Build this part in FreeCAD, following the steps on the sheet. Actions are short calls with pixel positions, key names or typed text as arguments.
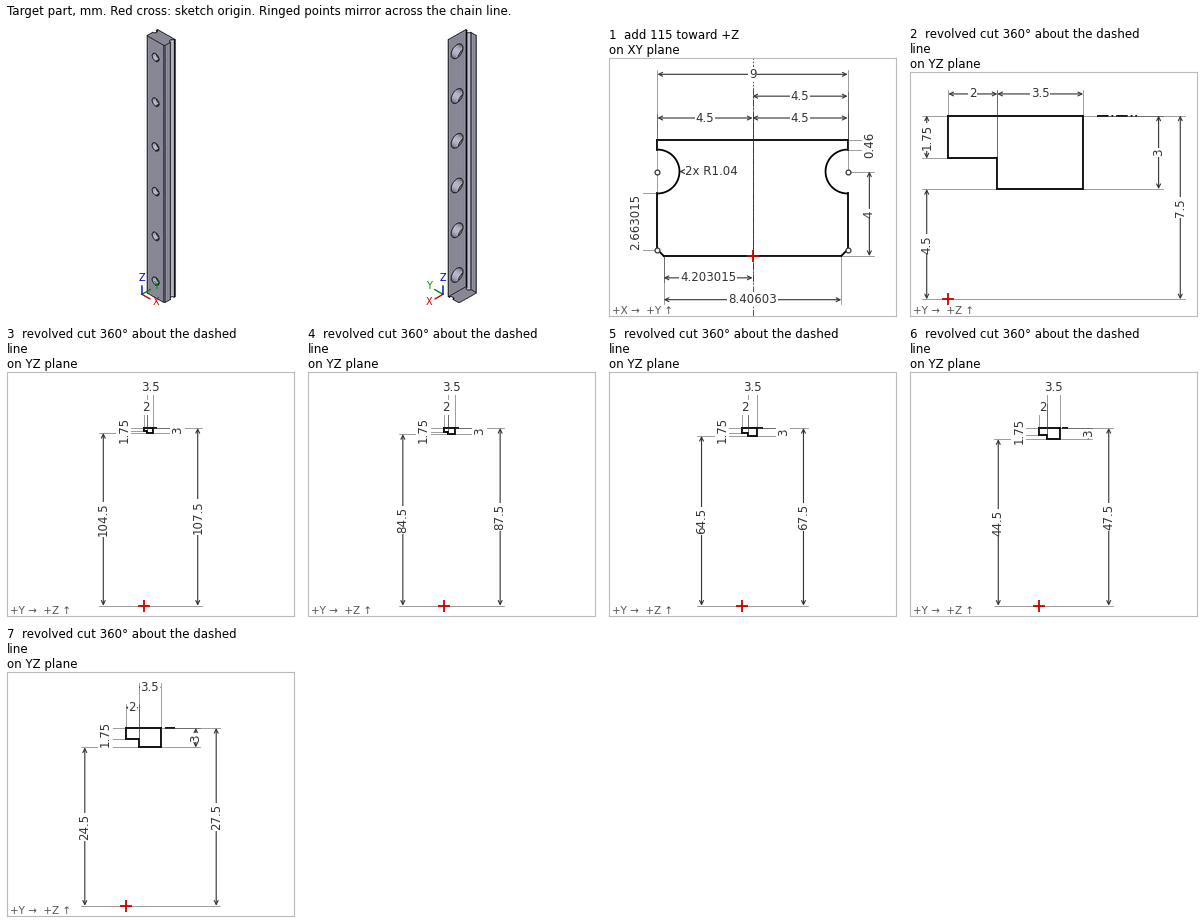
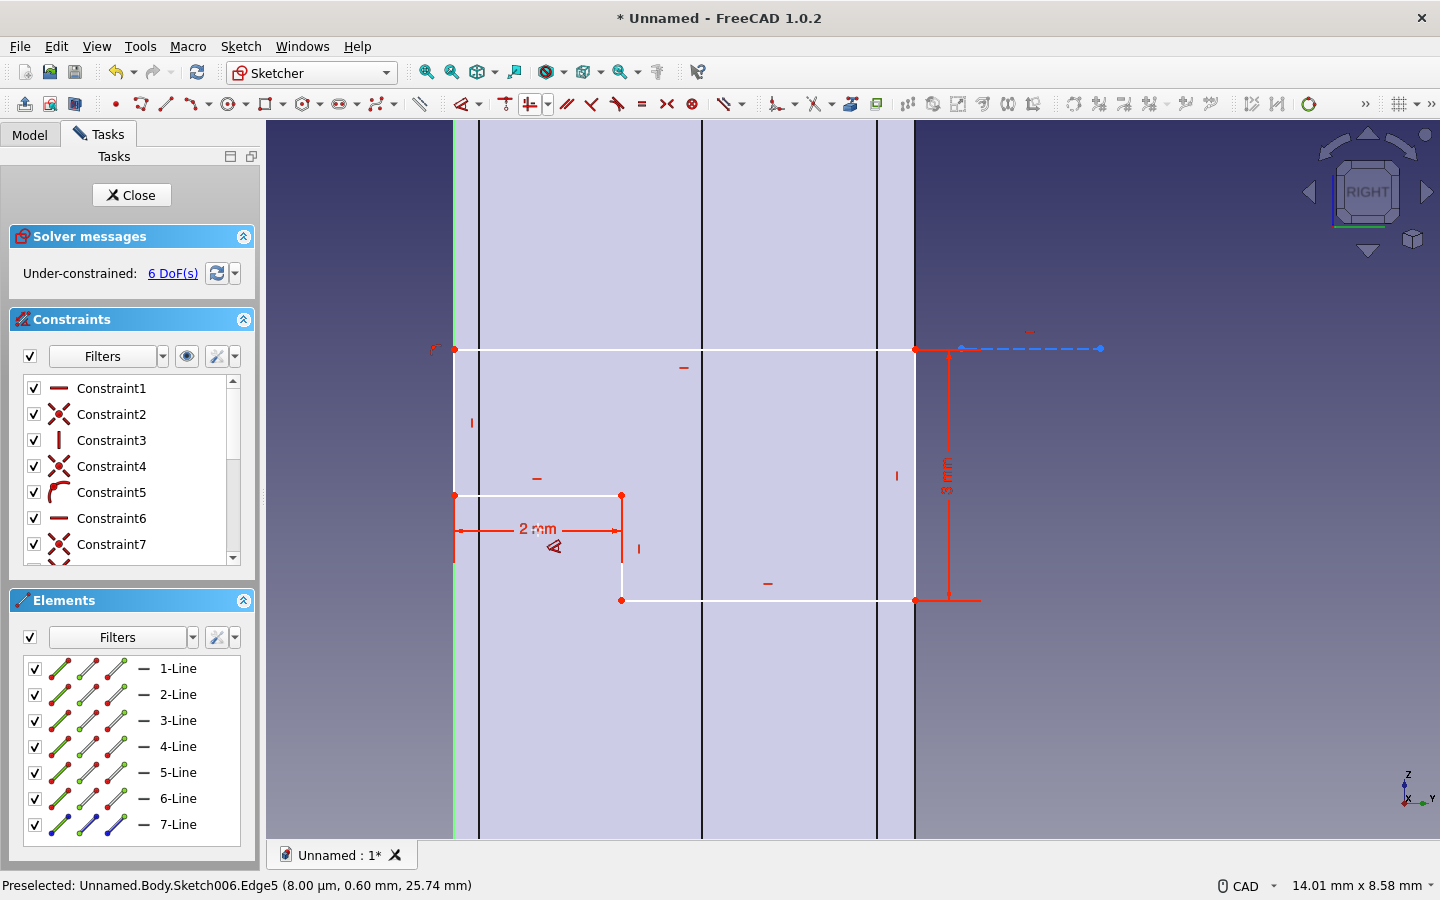
click(710, 601)
click(768, 635)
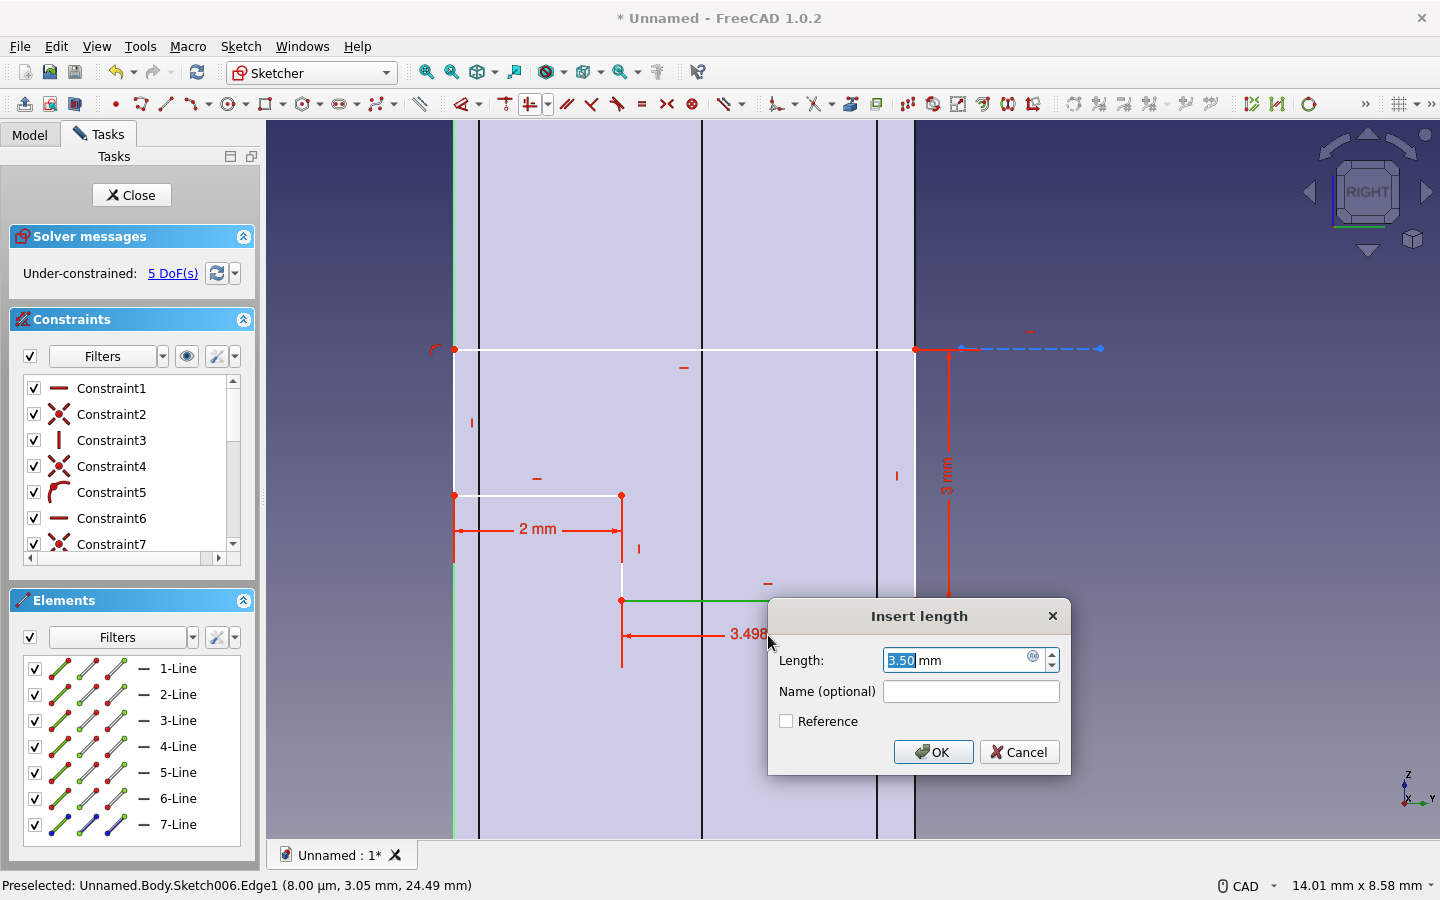
text(3.5)
key(Return)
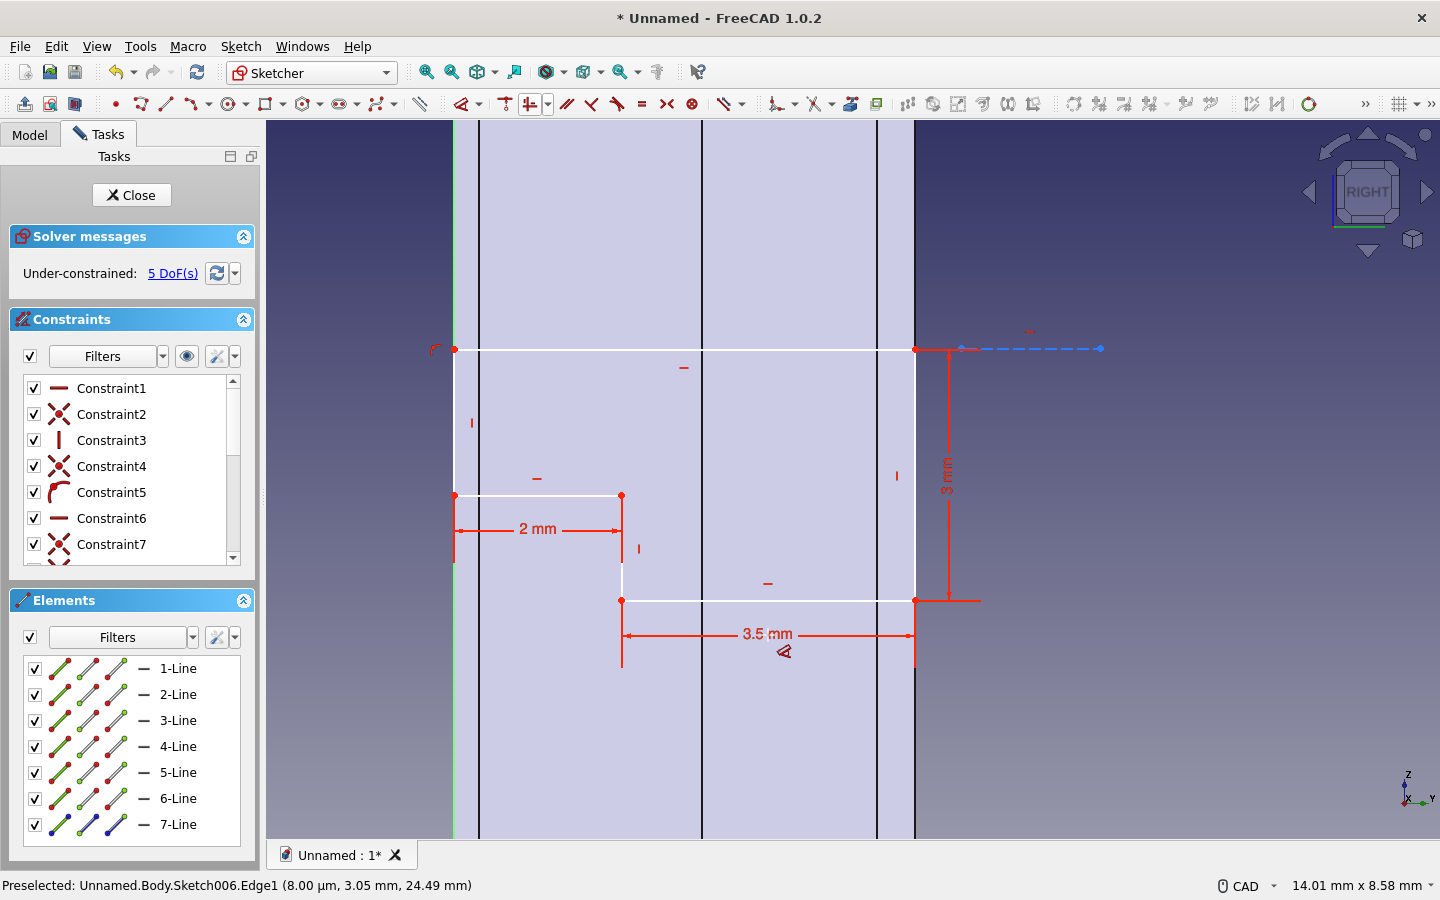
click(454, 393)
click(420, 423)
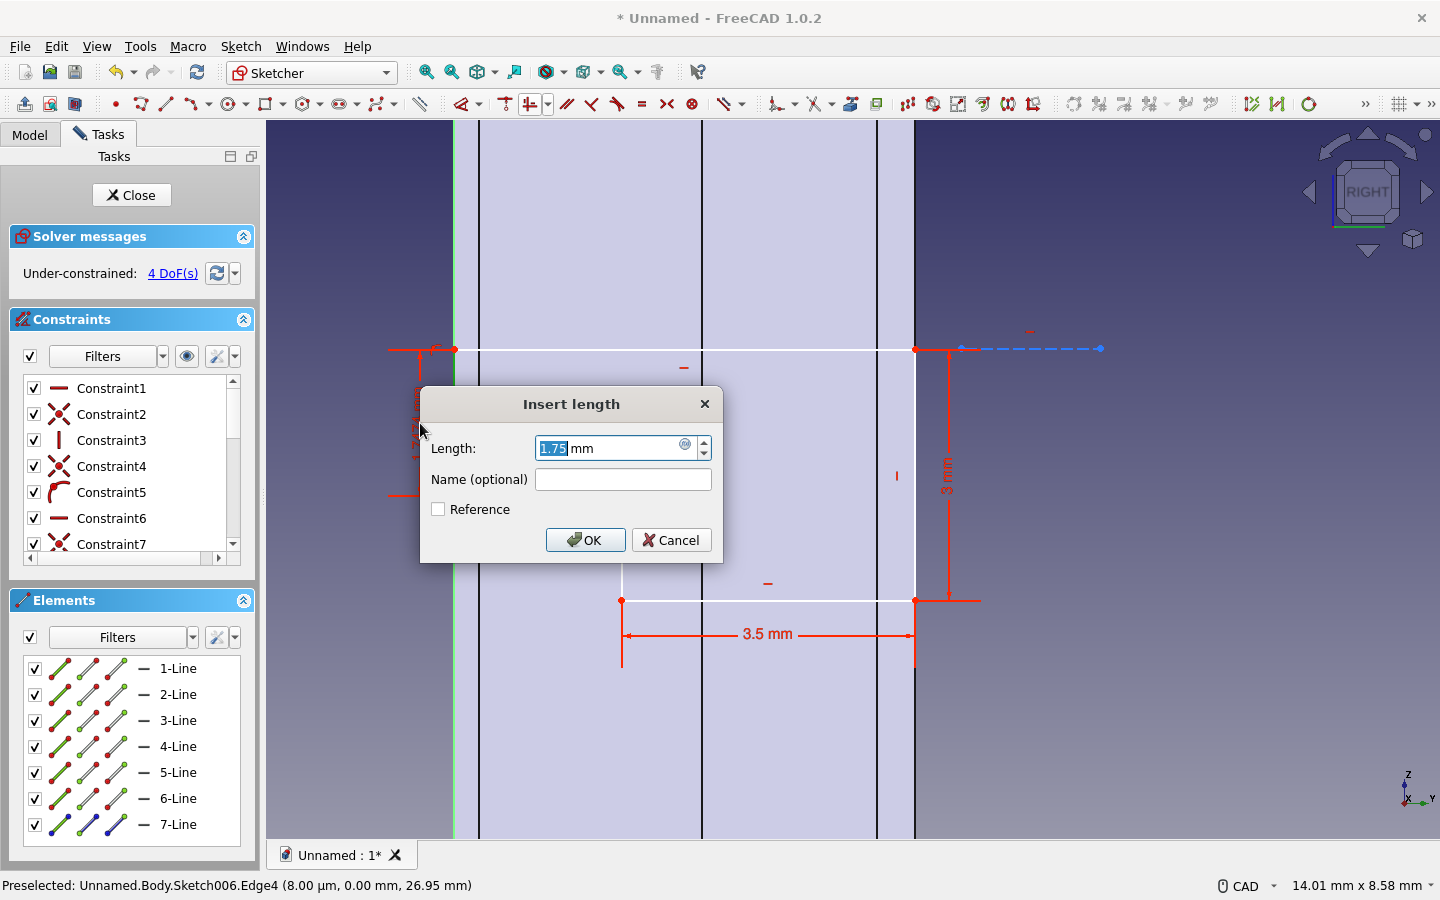
text(1.75)
key(Return)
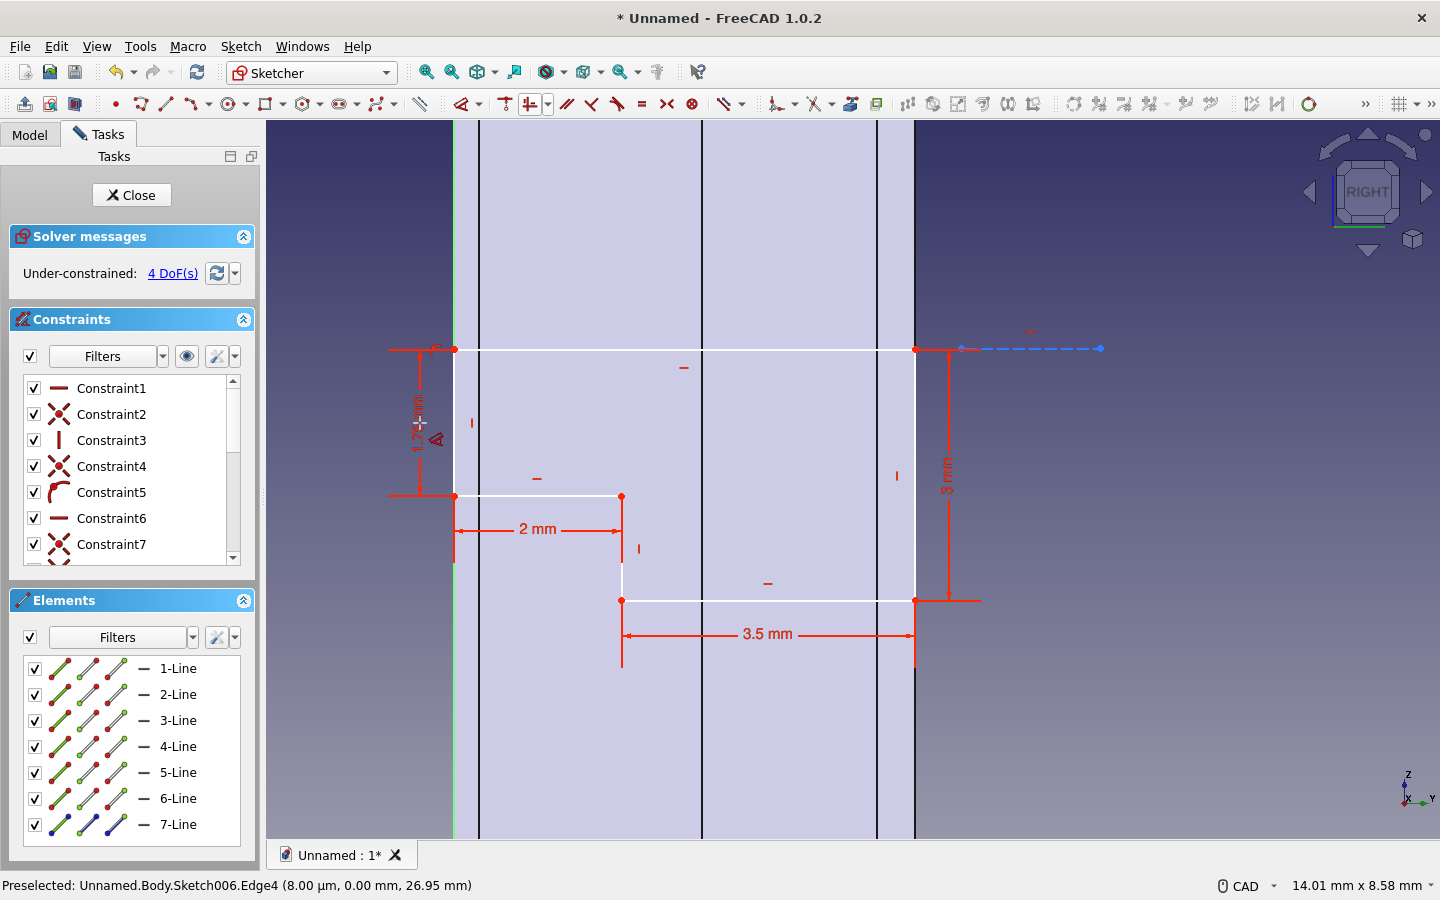
click(622, 601)
click(420, 706)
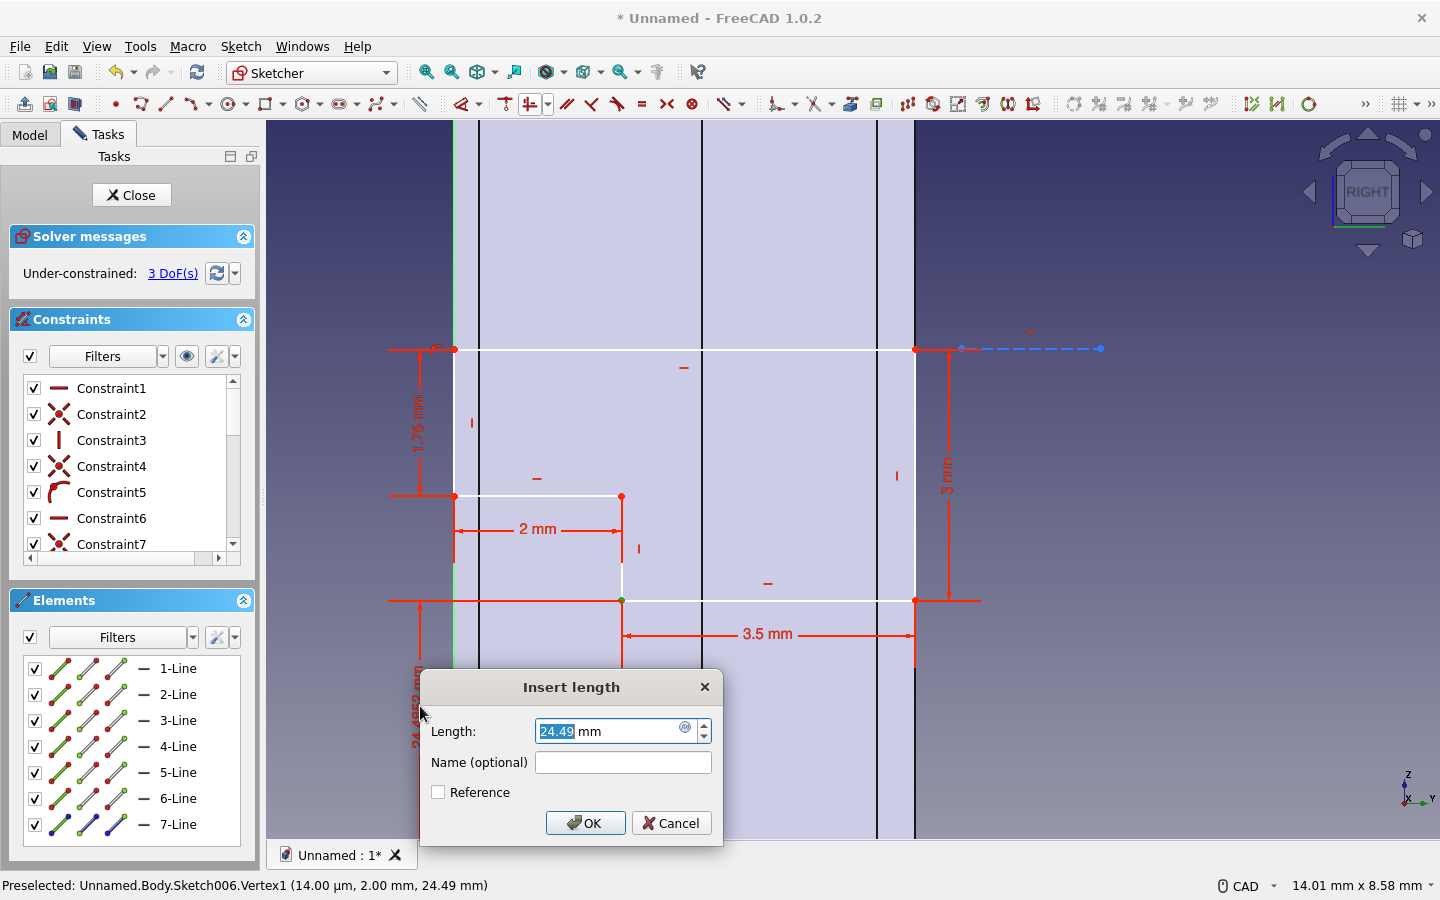
text(24.5)
key(Return)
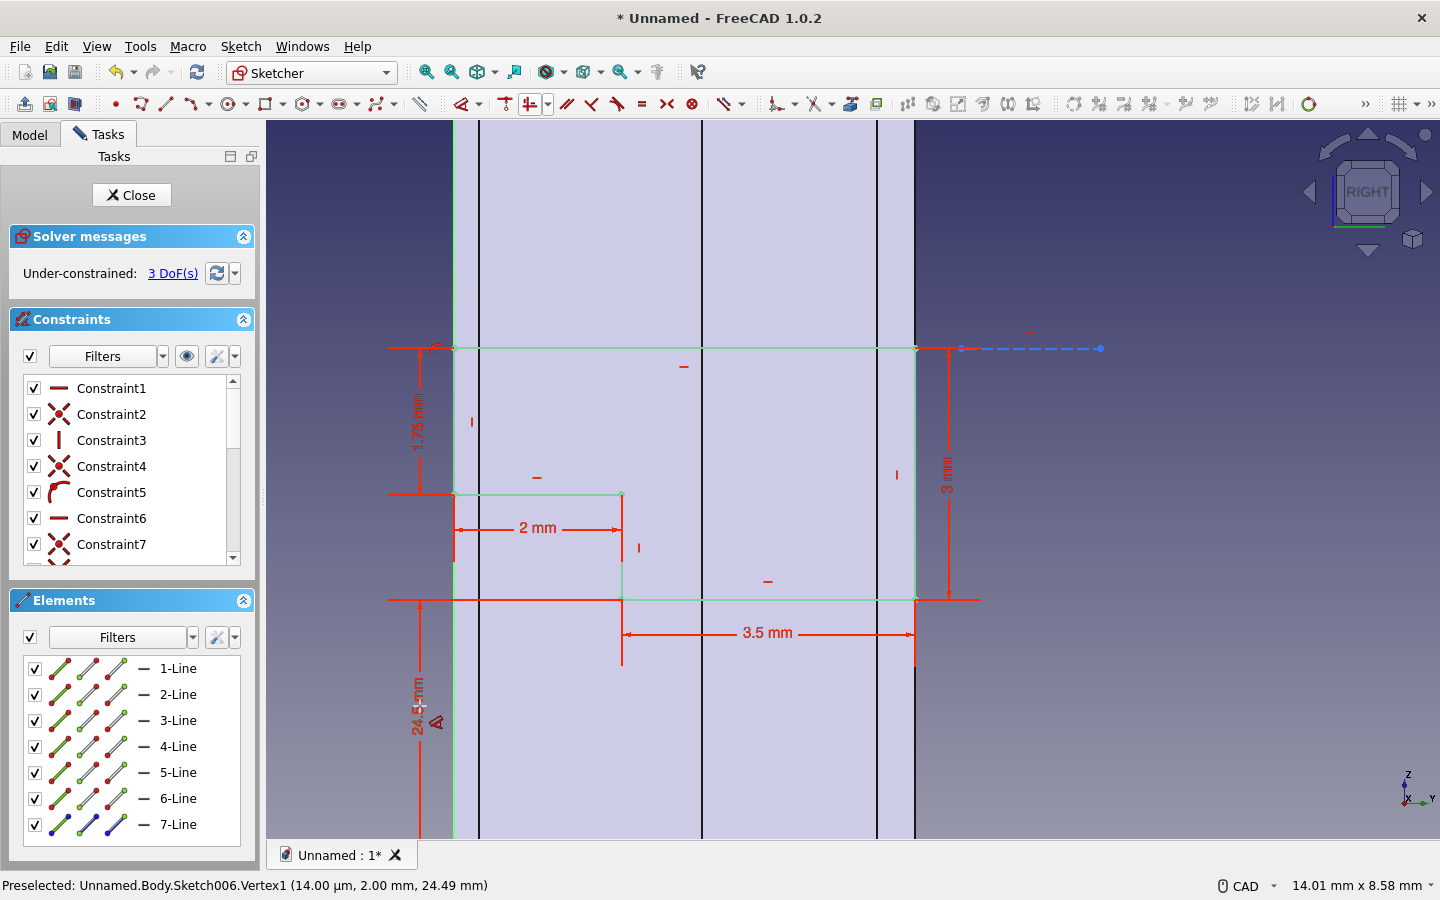
click(961, 349)
click(420, 580)